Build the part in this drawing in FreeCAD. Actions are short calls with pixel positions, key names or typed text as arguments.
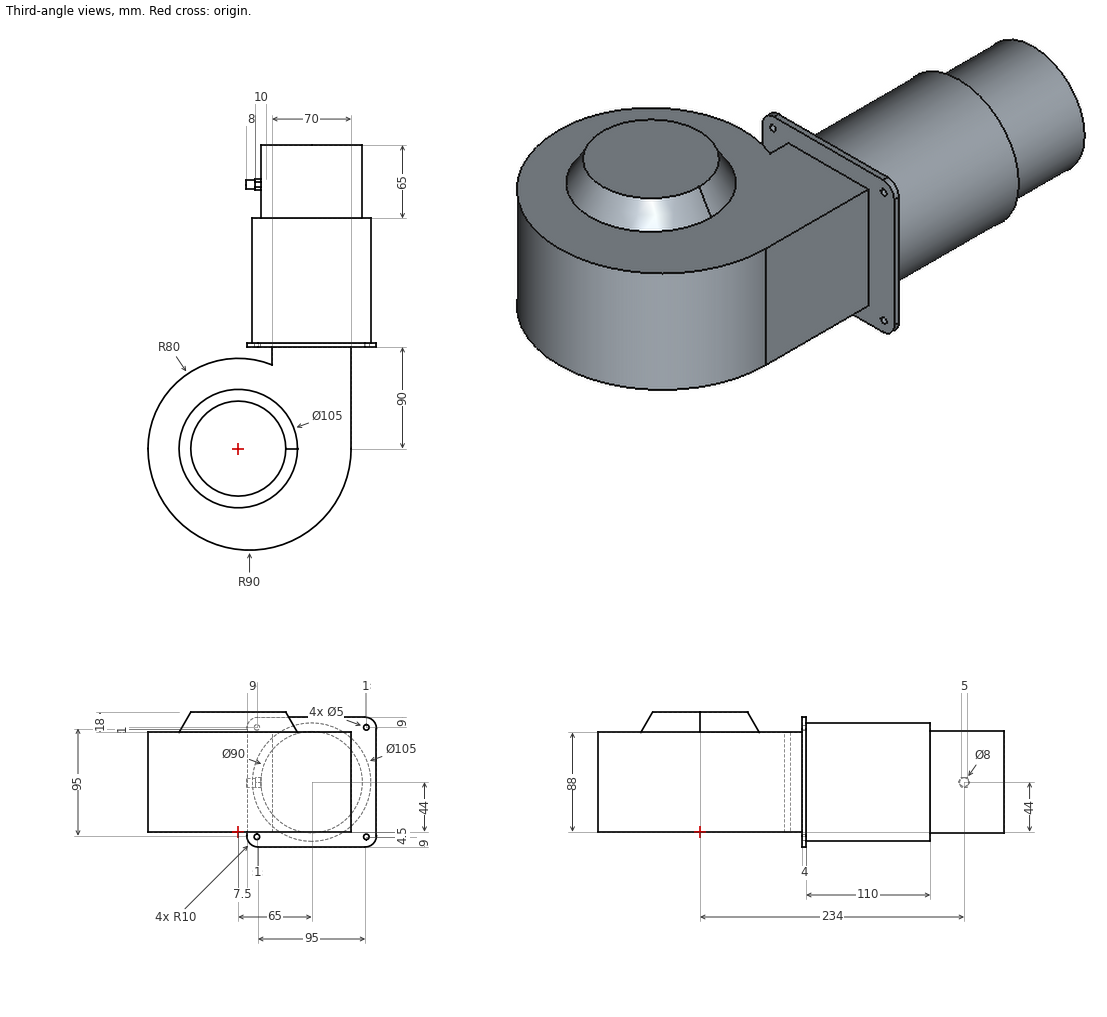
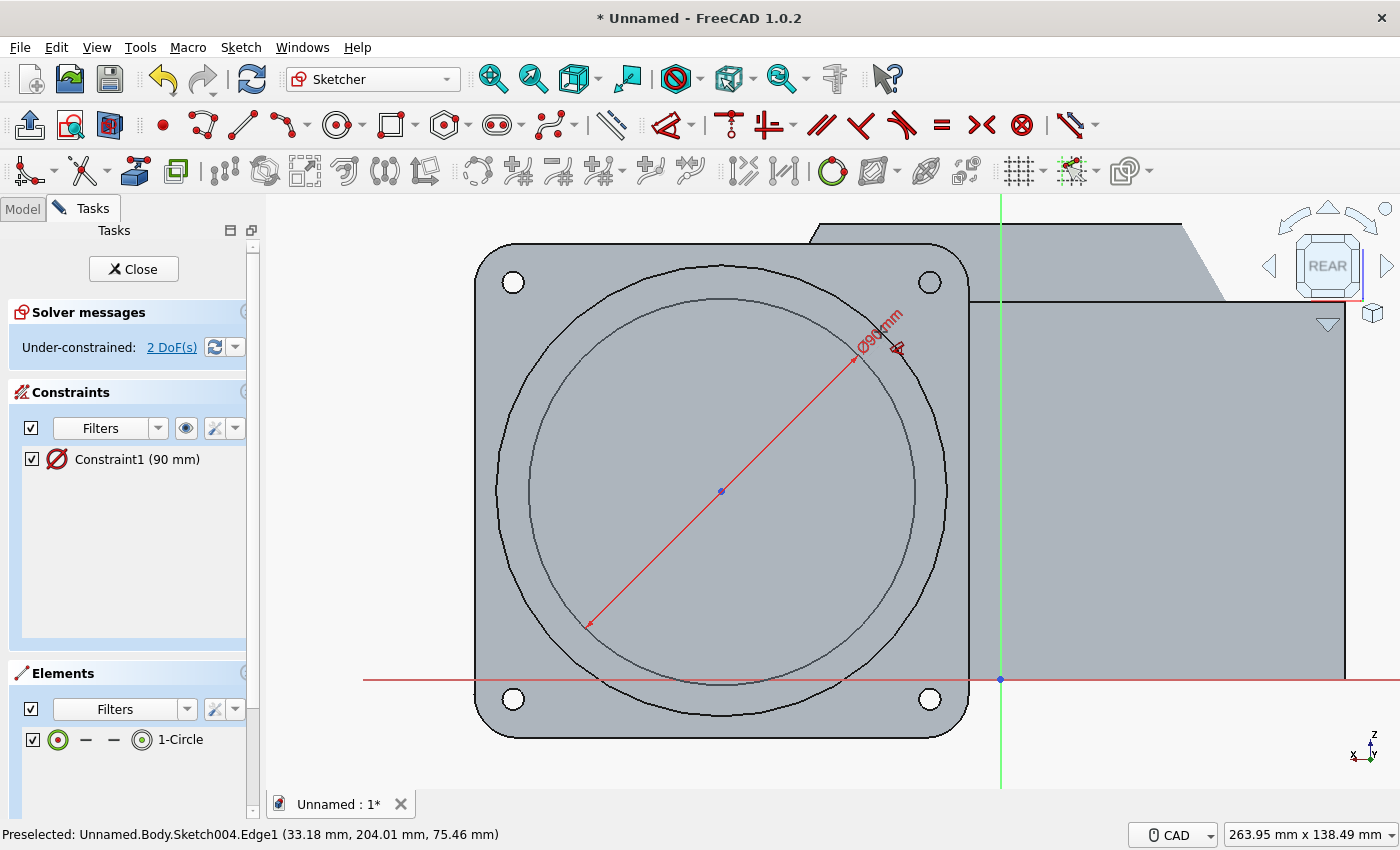
click(722, 492)
click(861, 714)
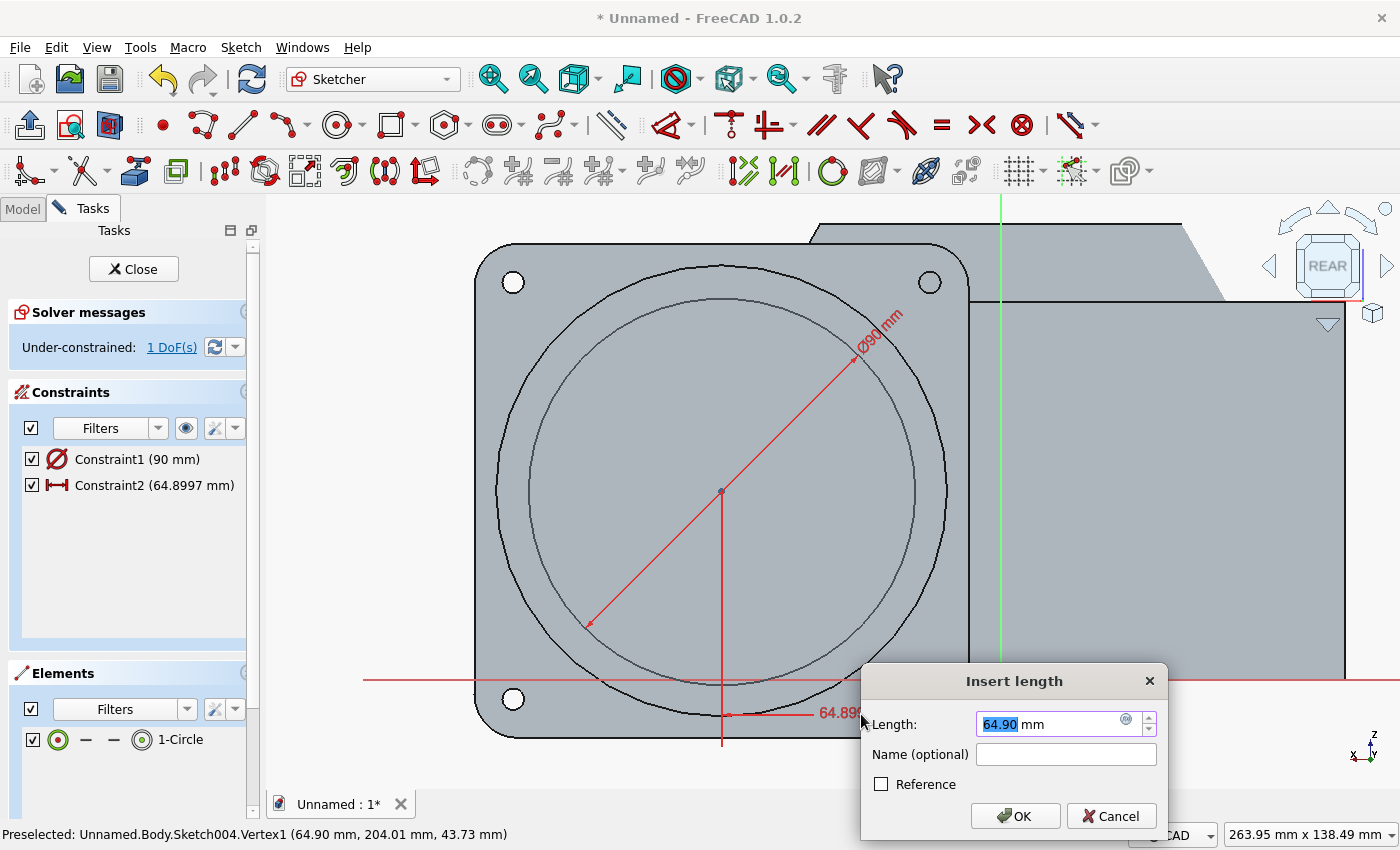
text(65)
key(Return)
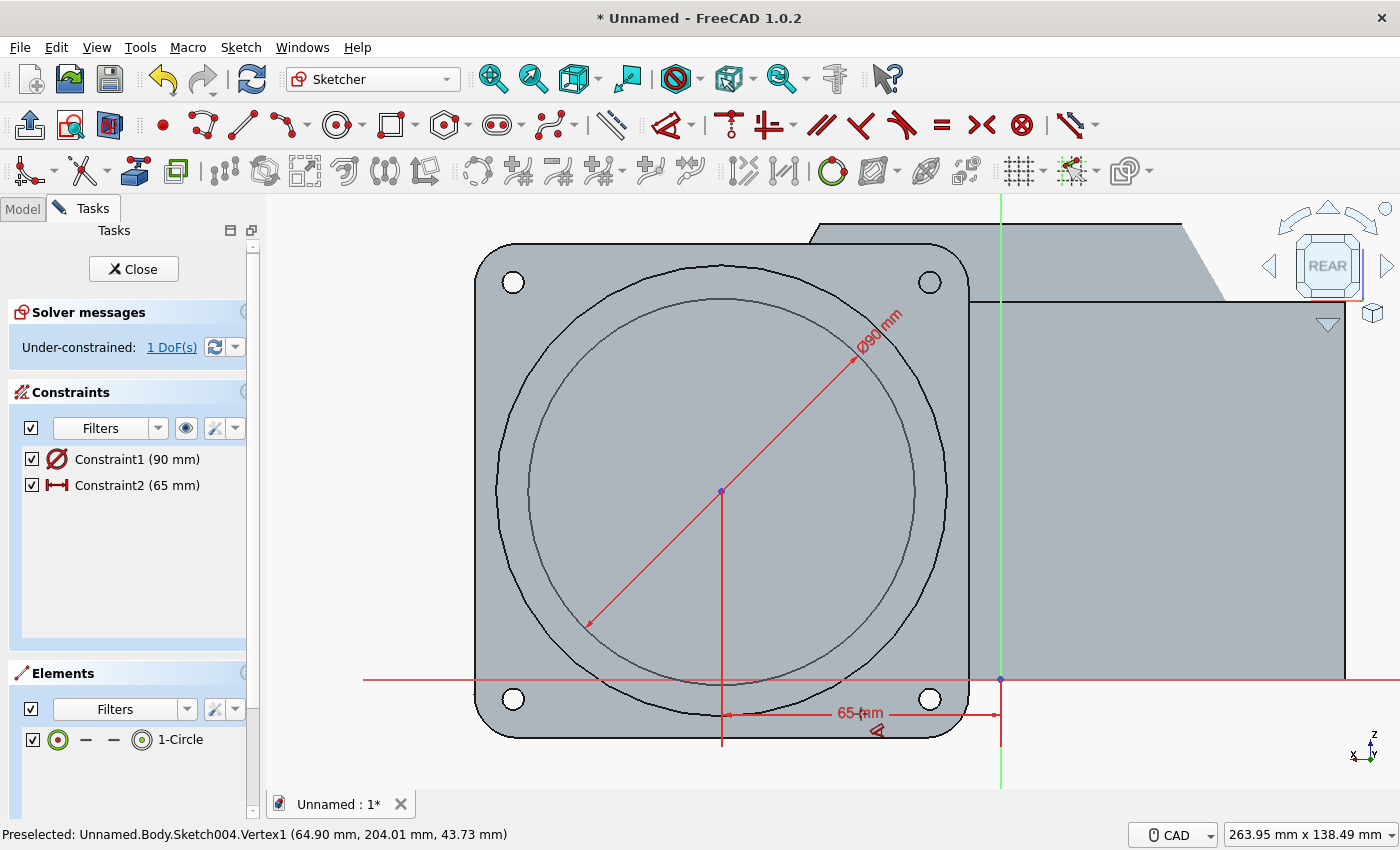
click(722, 492)
click(1035, 586)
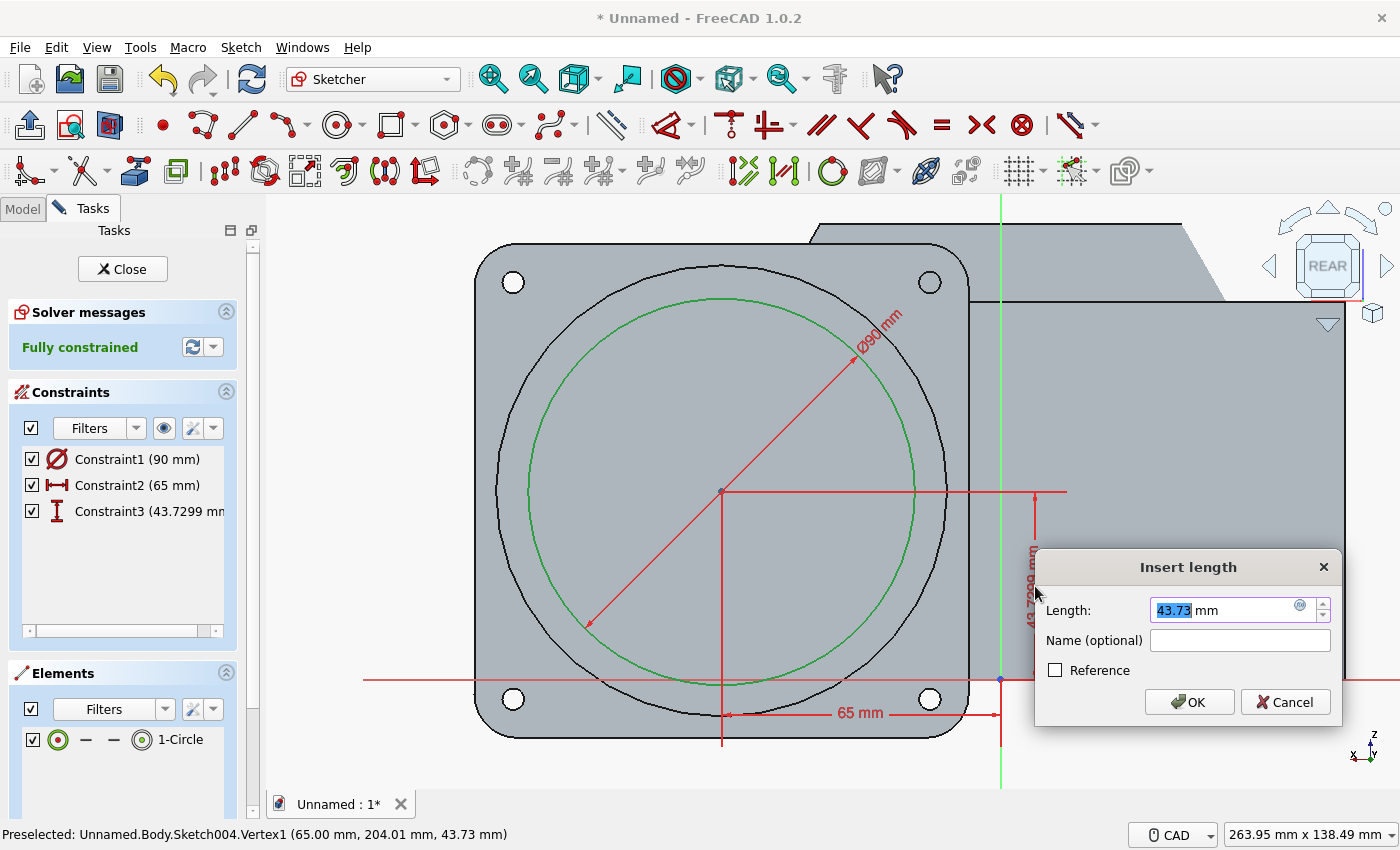
text(44)
key(Return)
key(Escape)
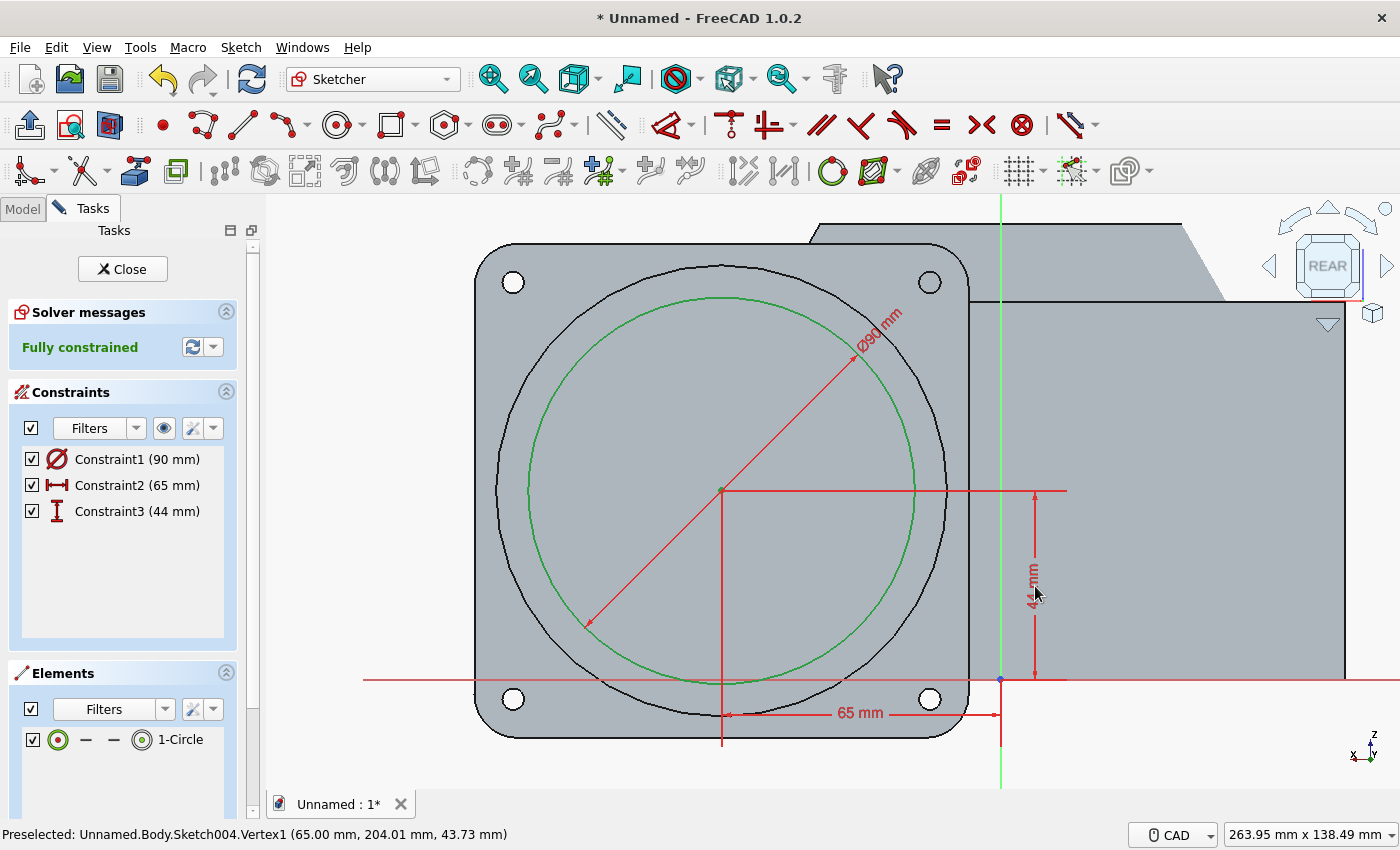
click(123, 269)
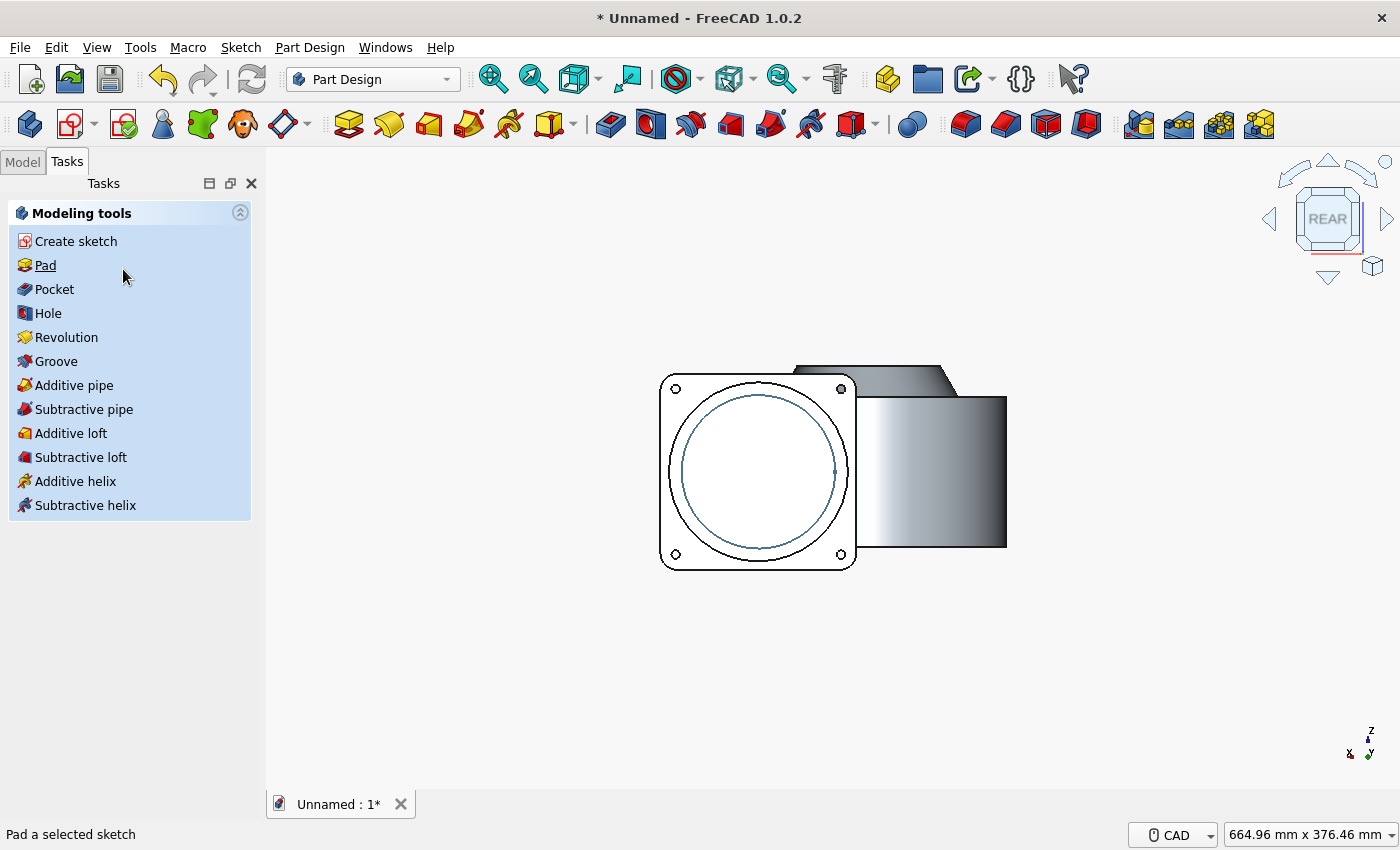
click(350, 124)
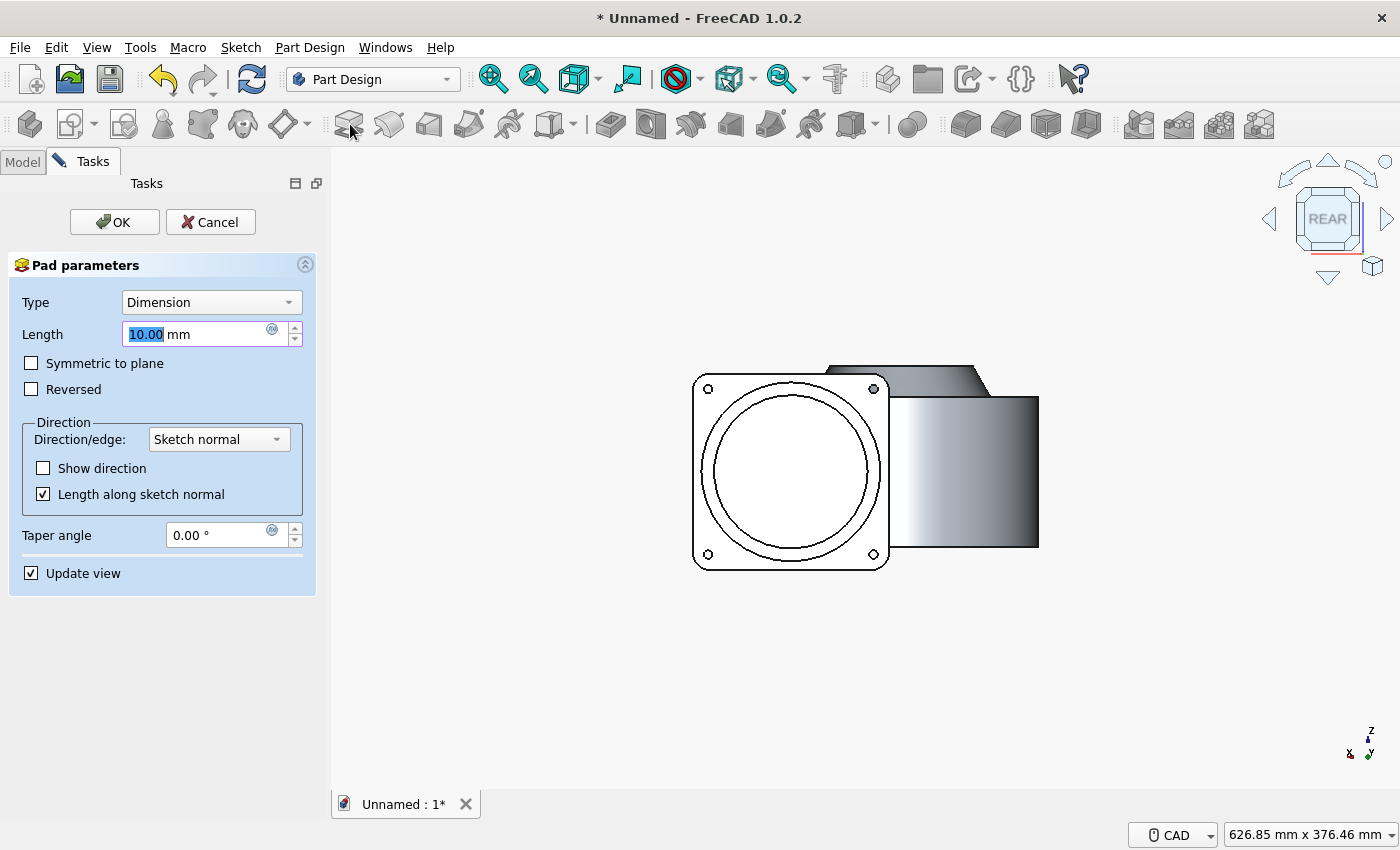
text(65)
key(Tab)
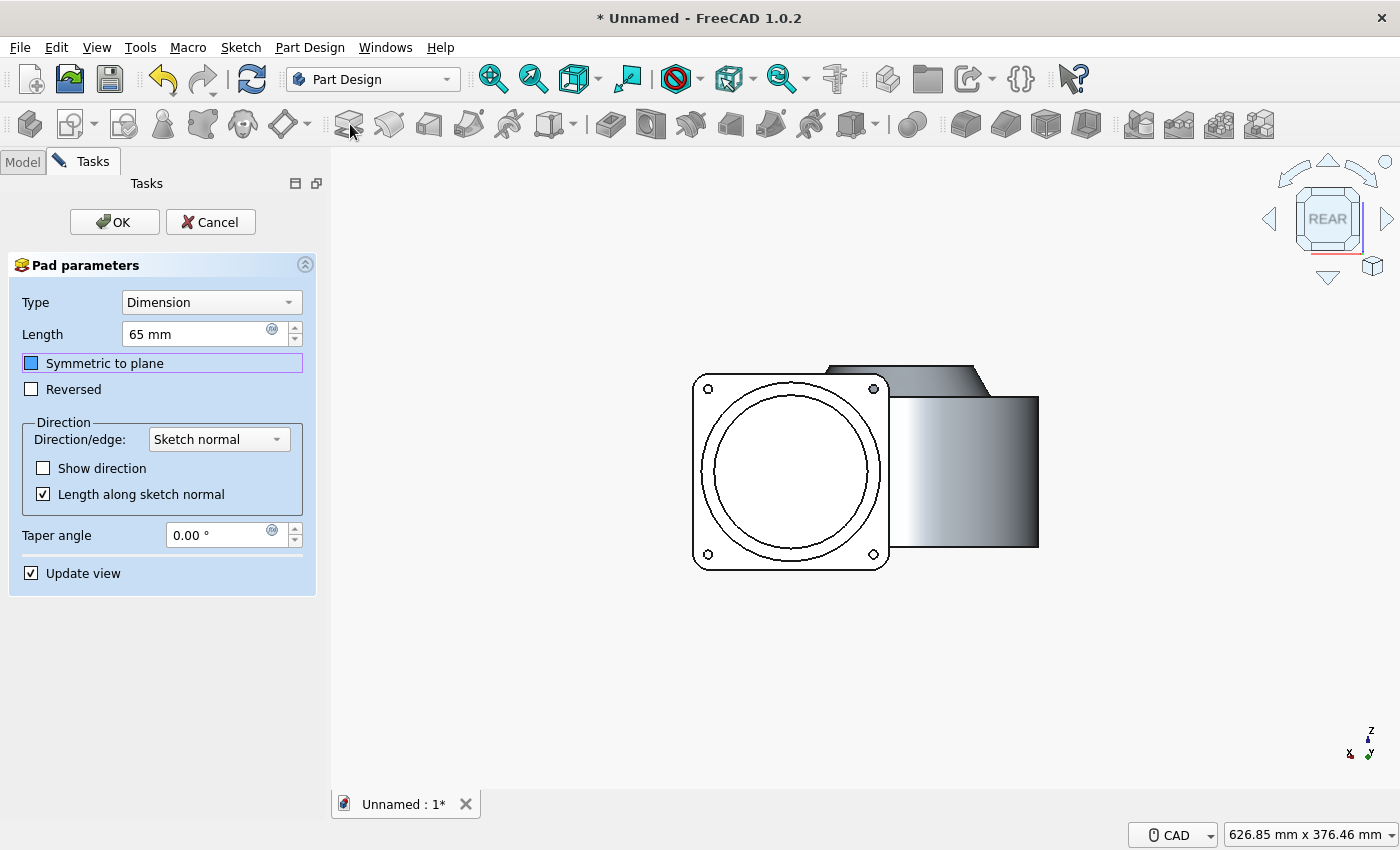
click(115, 222)